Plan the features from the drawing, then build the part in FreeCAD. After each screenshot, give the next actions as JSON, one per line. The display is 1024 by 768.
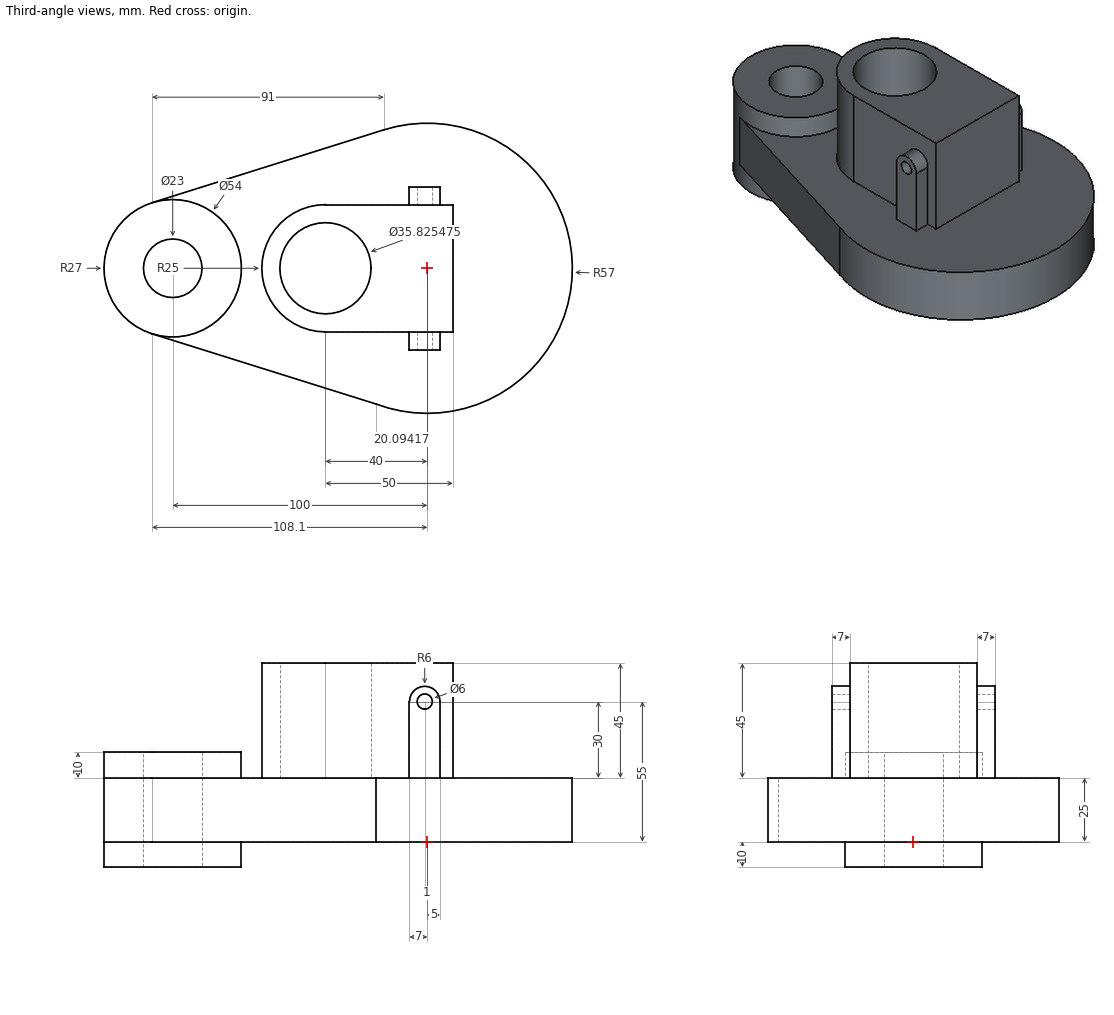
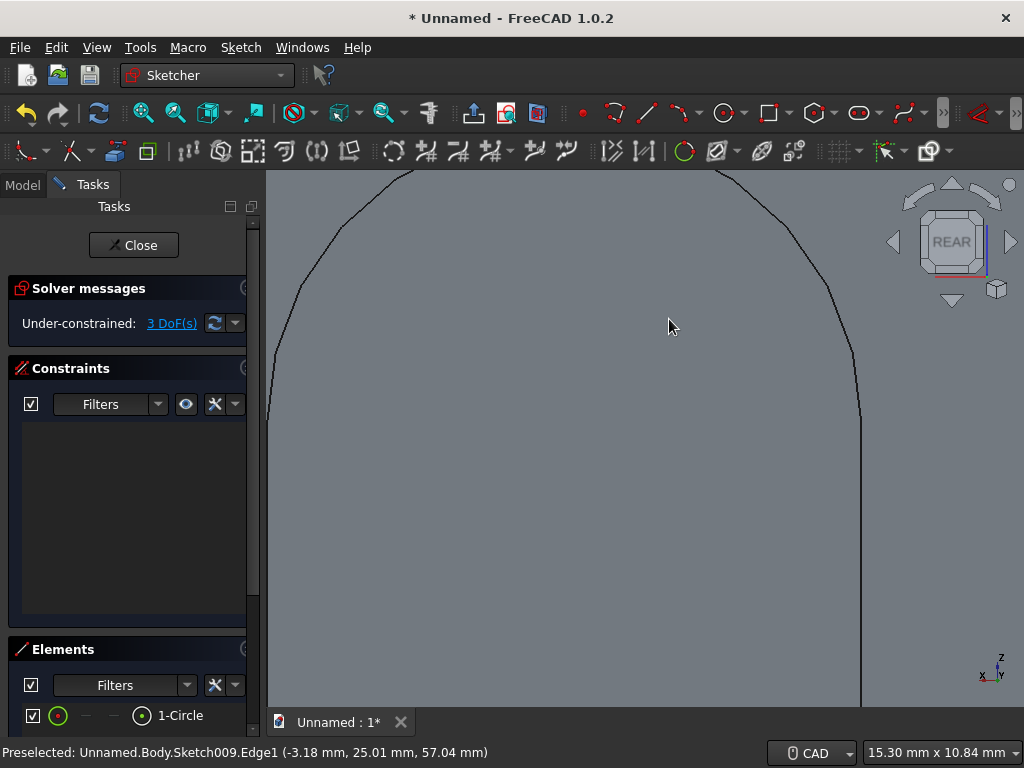
{"action": "left_click", "coordinate": [978, 114]}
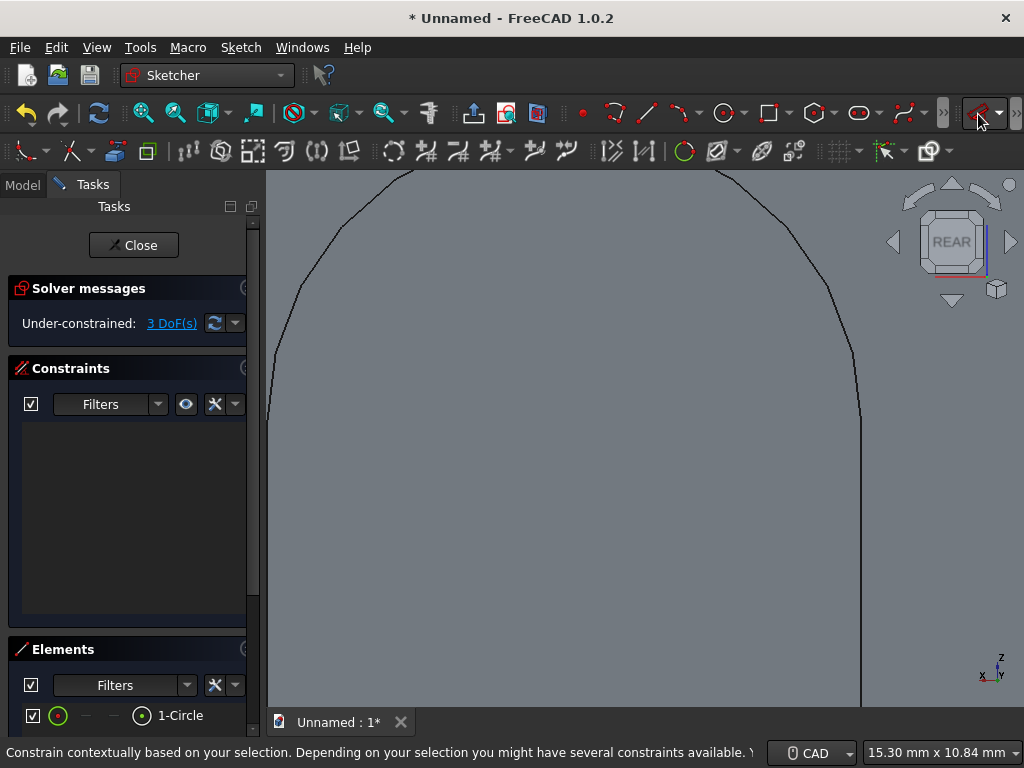
{"action": "left_click", "coordinate": [669, 320]}
{"action": "left_click", "coordinate": [692, 297]}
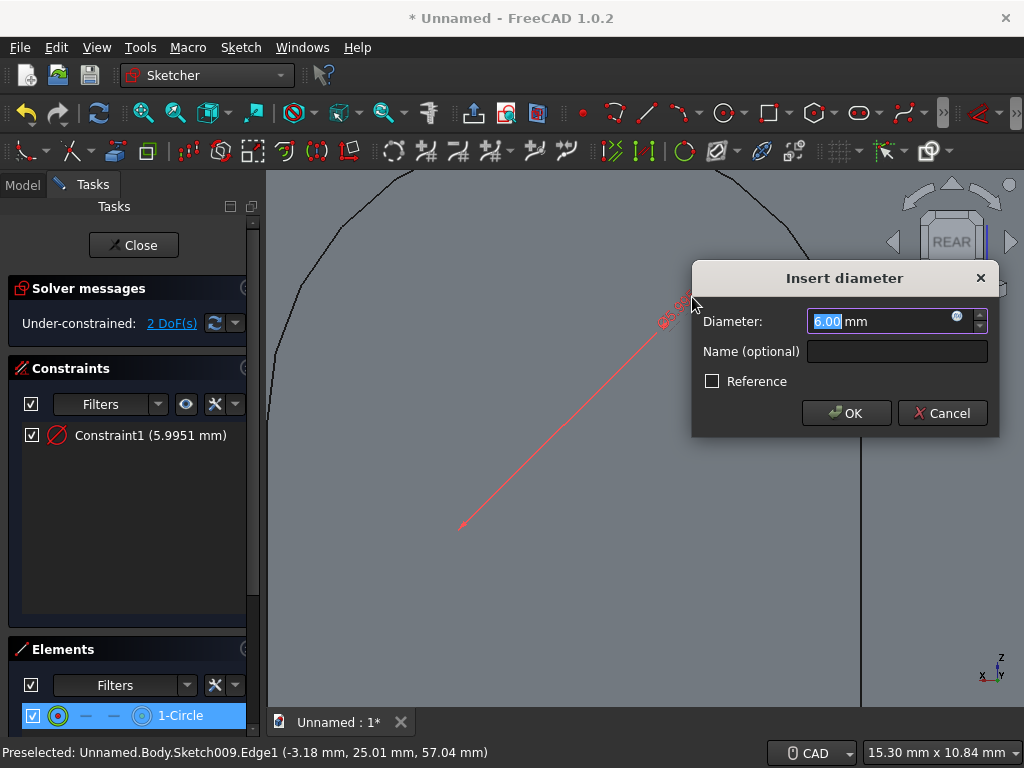
{"action": "type", "text": "6"}
{"action": "key", "text": "Return"}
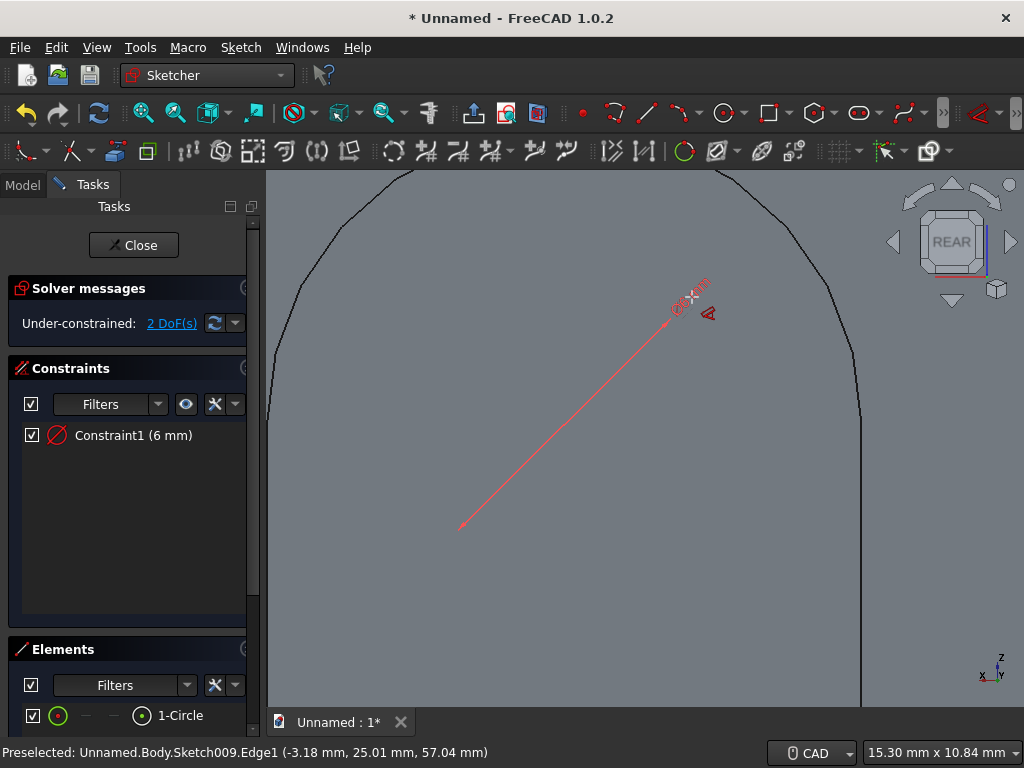
{"action": "left_click", "coordinate": [564, 425]}
{"action": "left_click", "coordinate": [539, 391]}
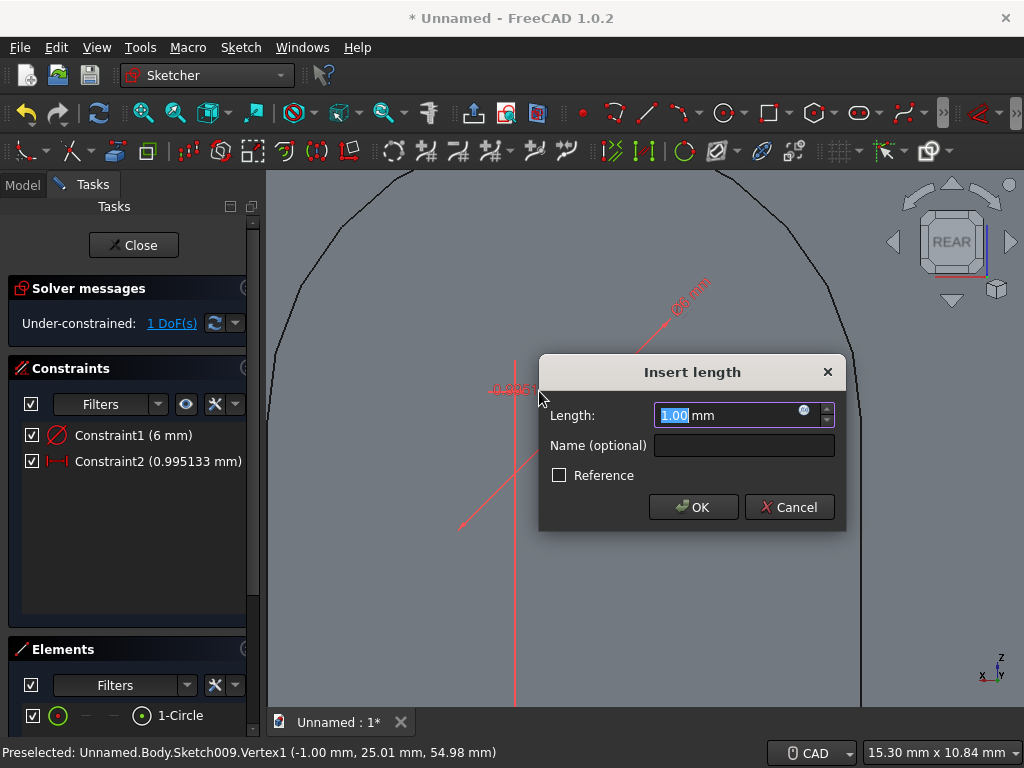
{"action": "type", "text": "1"}
{"action": "key", "text": "Return"}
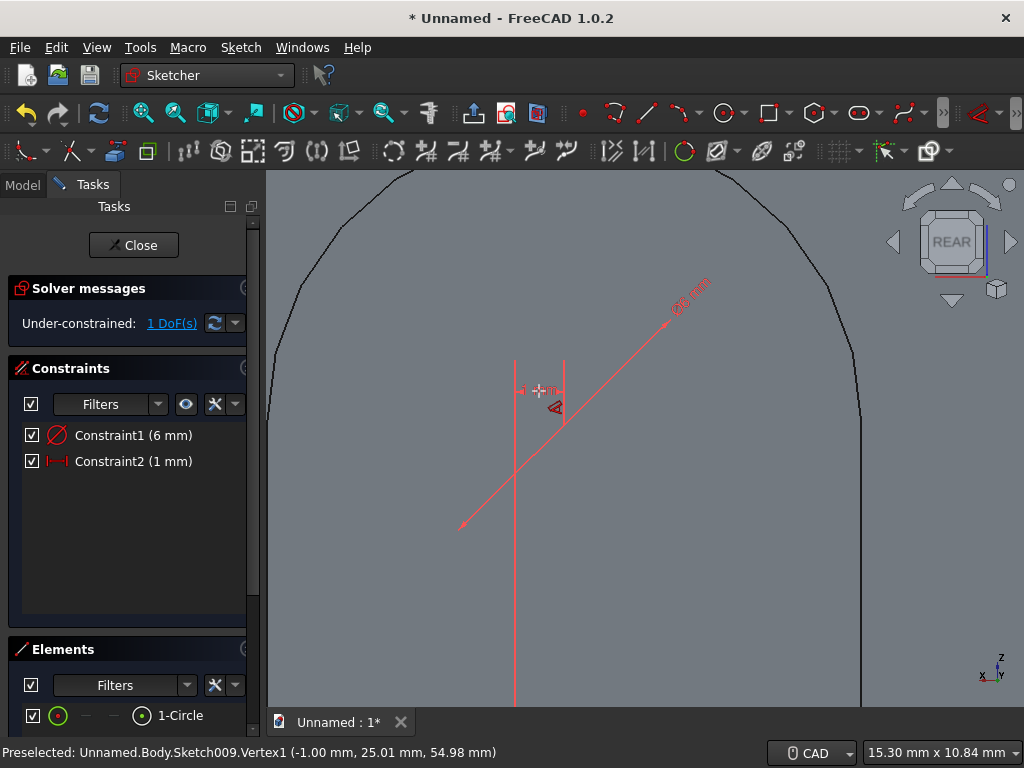
{"action": "left_click", "coordinate": [564, 425]}
{"action": "left_click", "coordinate": [481, 494]}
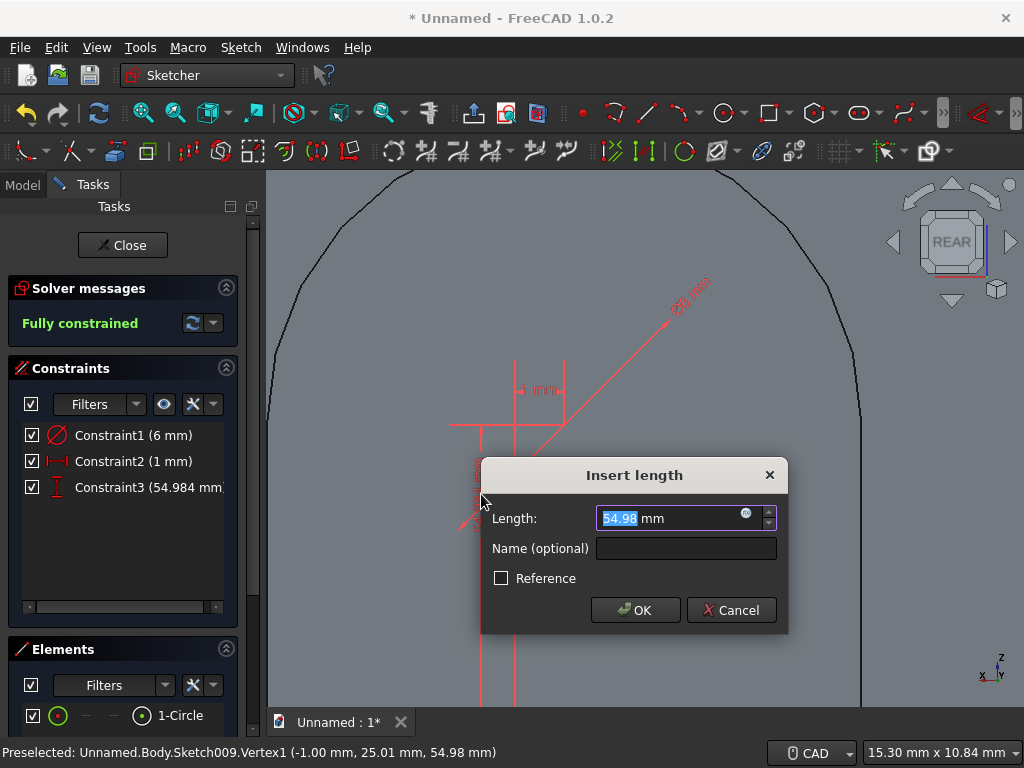
{"action": "type", "text": "55"}
{"action": "key", "text": "Return"}
{"action": "key", "text": "Escape"}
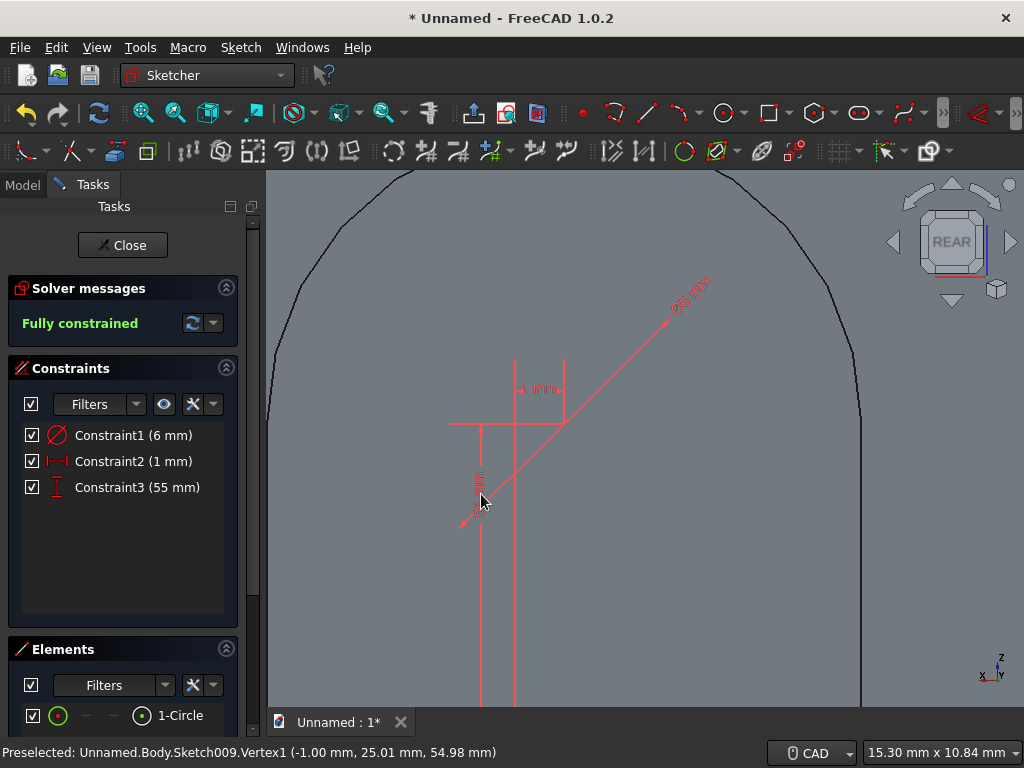
{"action": "left_click", "coordinate": [123, 245]}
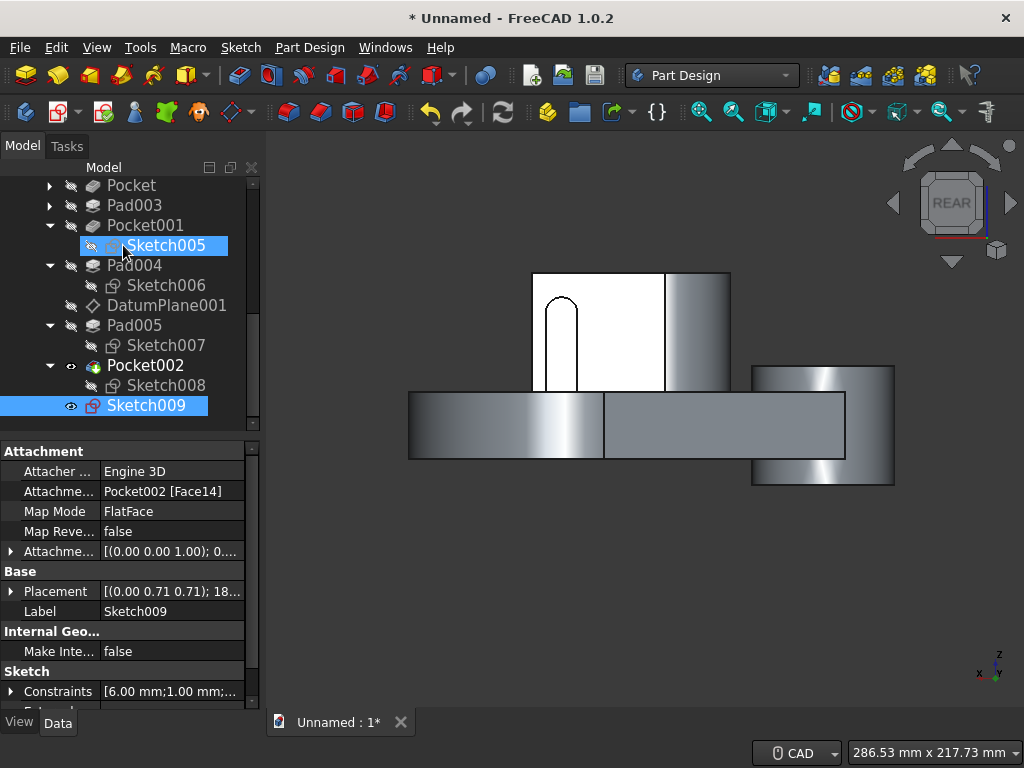
{"action": "left_click", "coordinate": [240, 76]}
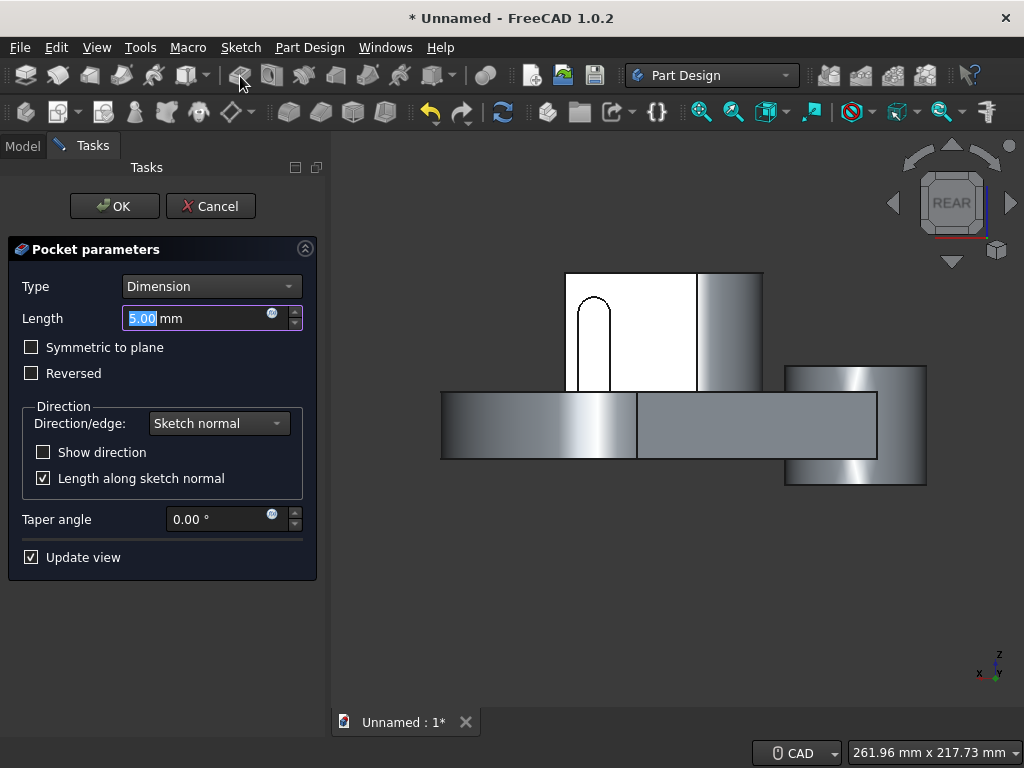
{"action": "type", "text": "7"}
{"action": "key", "text": "Tab"}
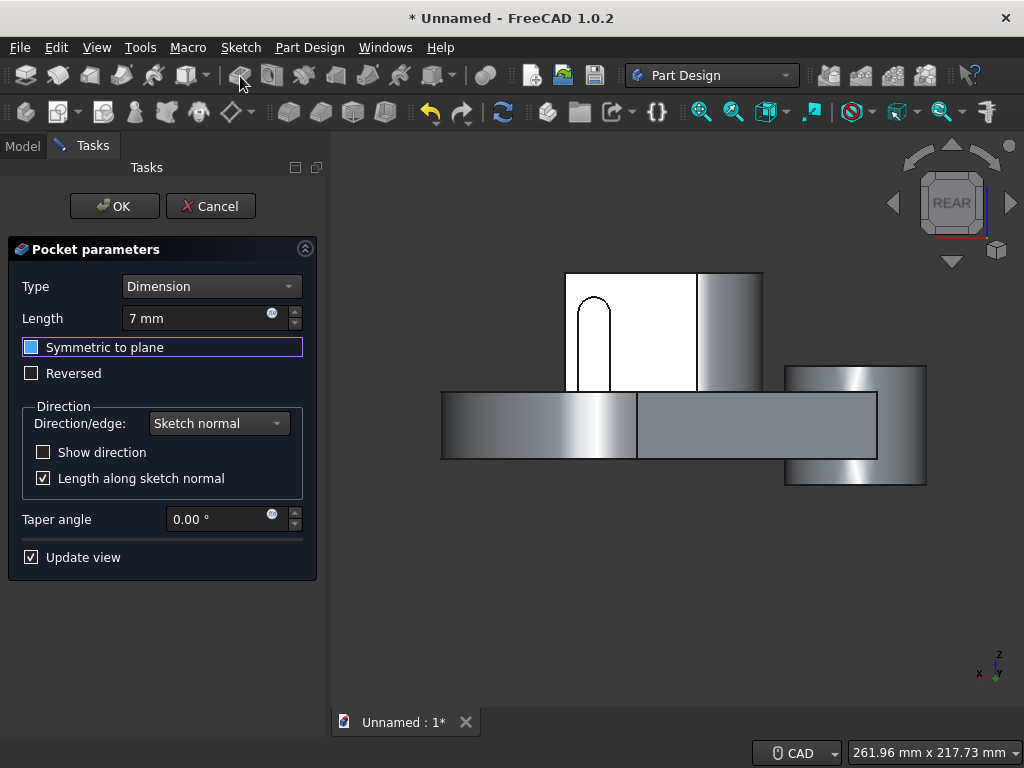
{"action": "left_click", "coordinate": [30, 373]}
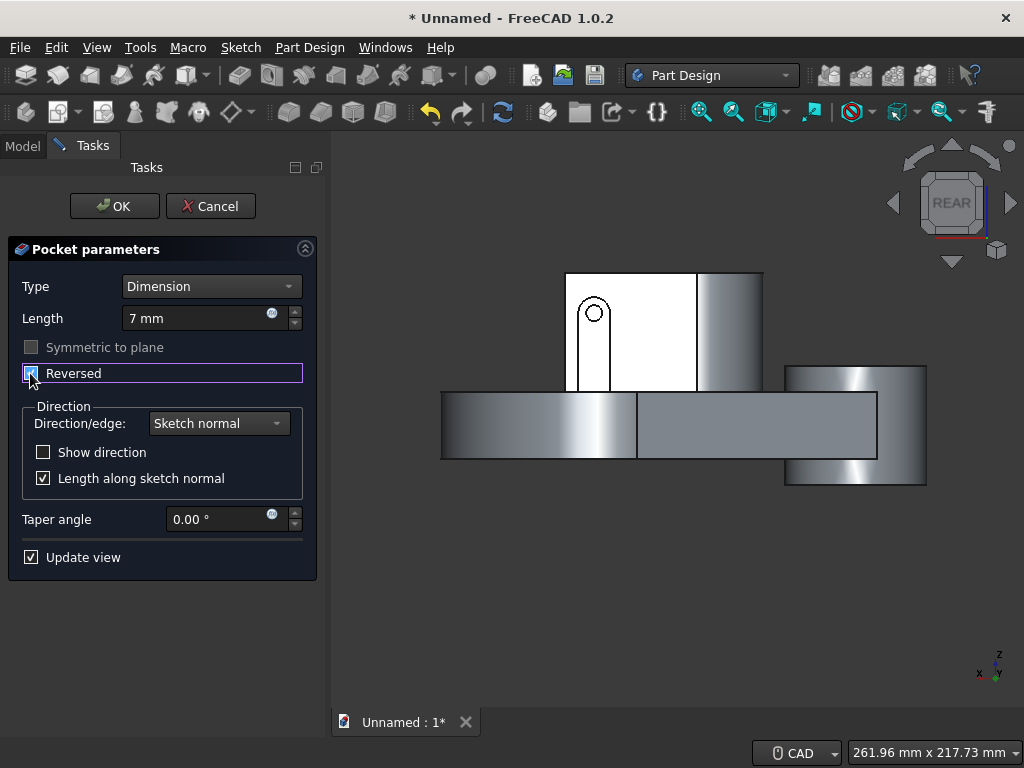
{"action": "left_click", "coordinate": [115, 206]}